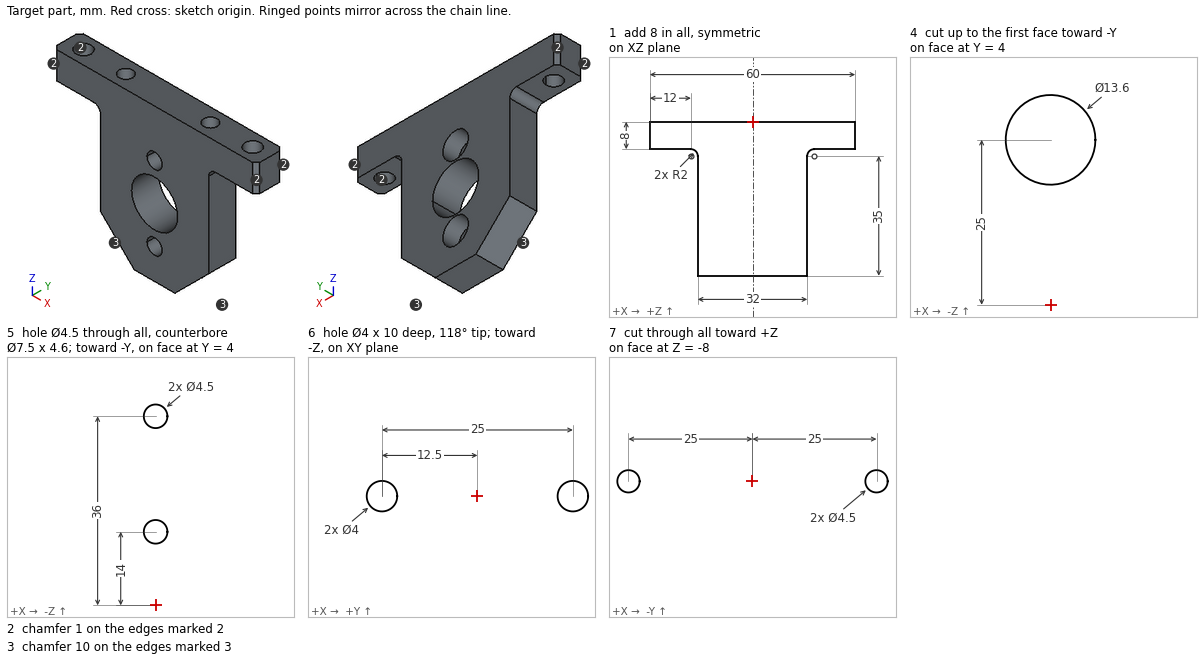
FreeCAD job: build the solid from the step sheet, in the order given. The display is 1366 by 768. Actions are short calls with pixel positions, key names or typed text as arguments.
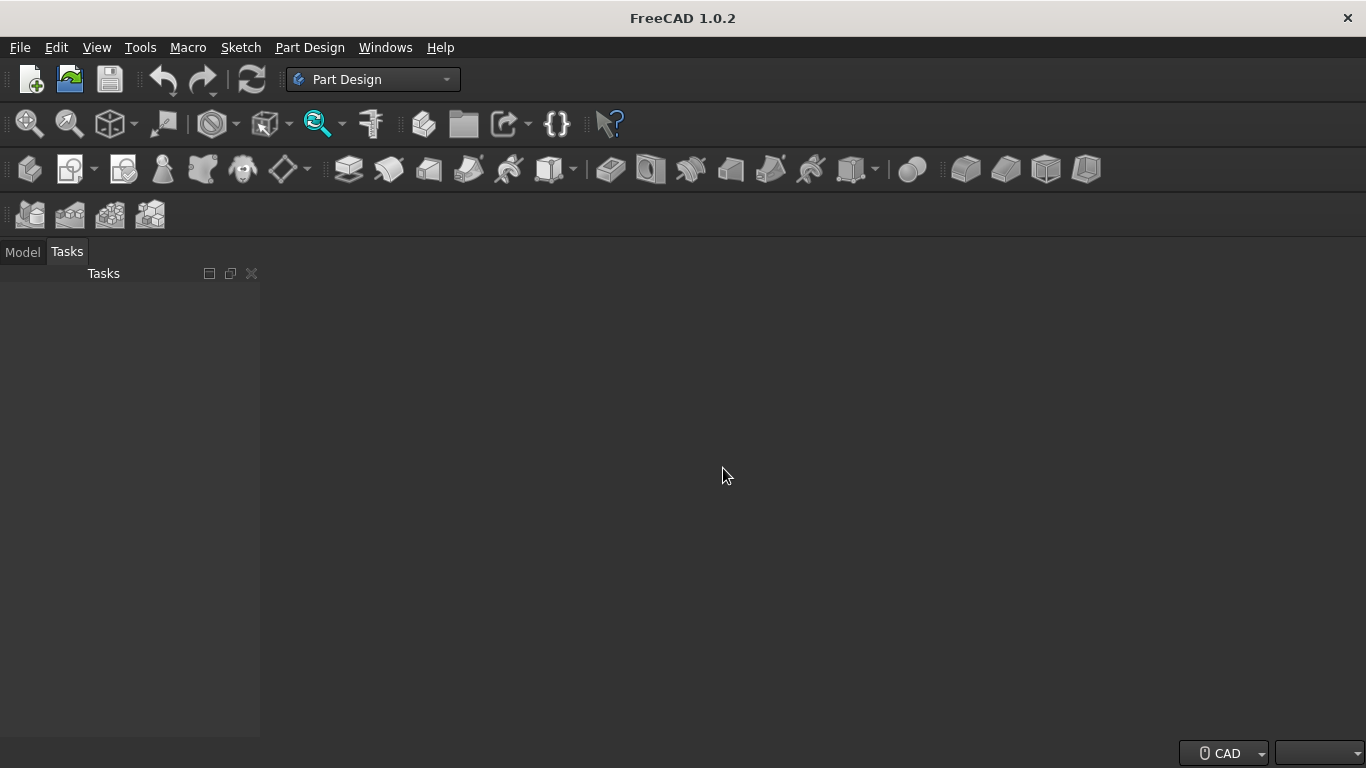
key(ctrl+n)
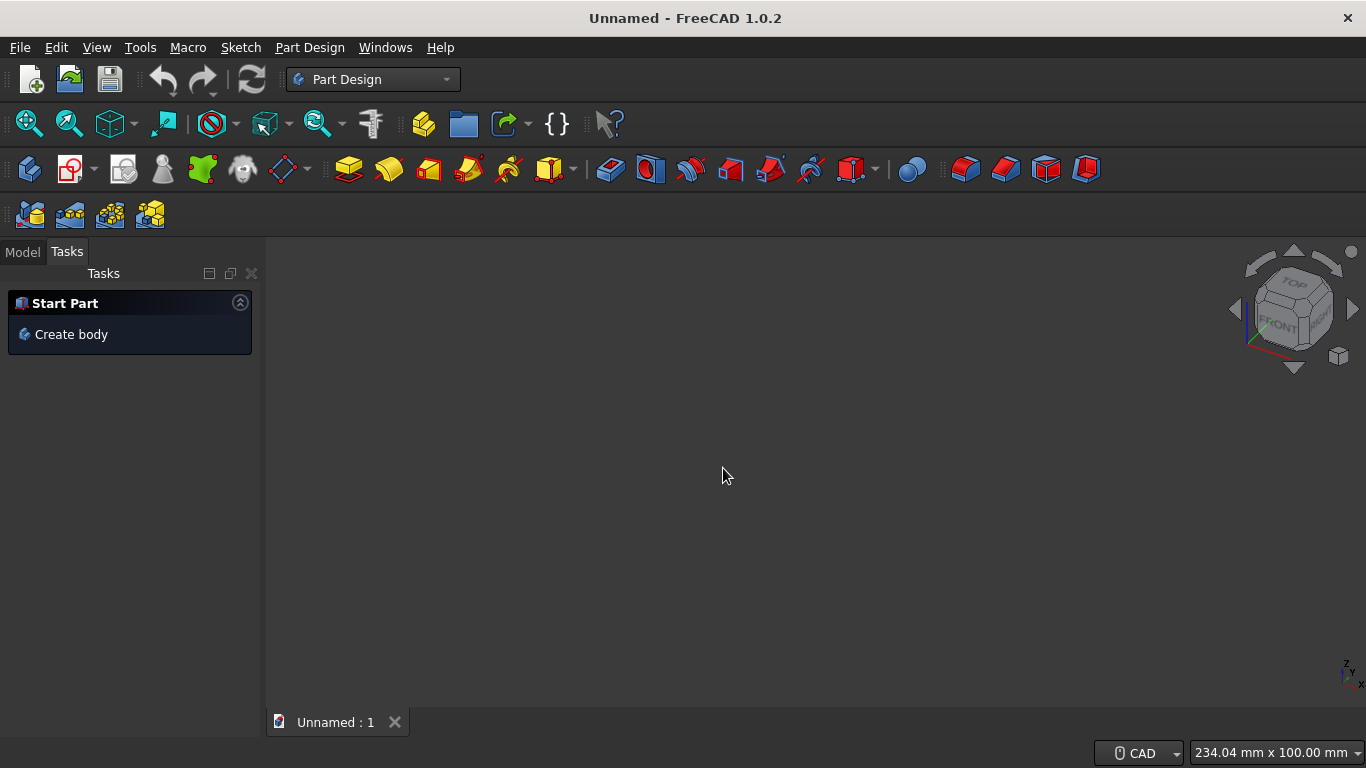
click(70, 170)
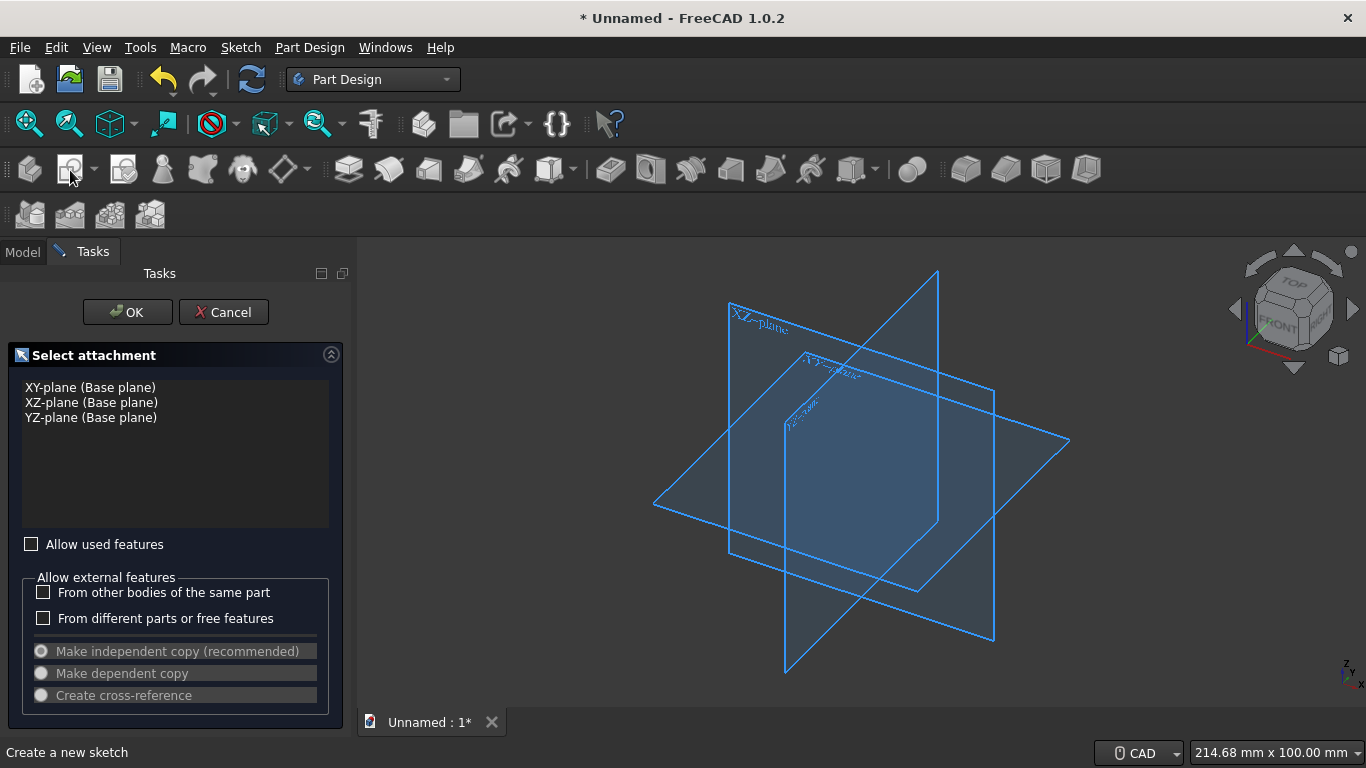
click(82, 402)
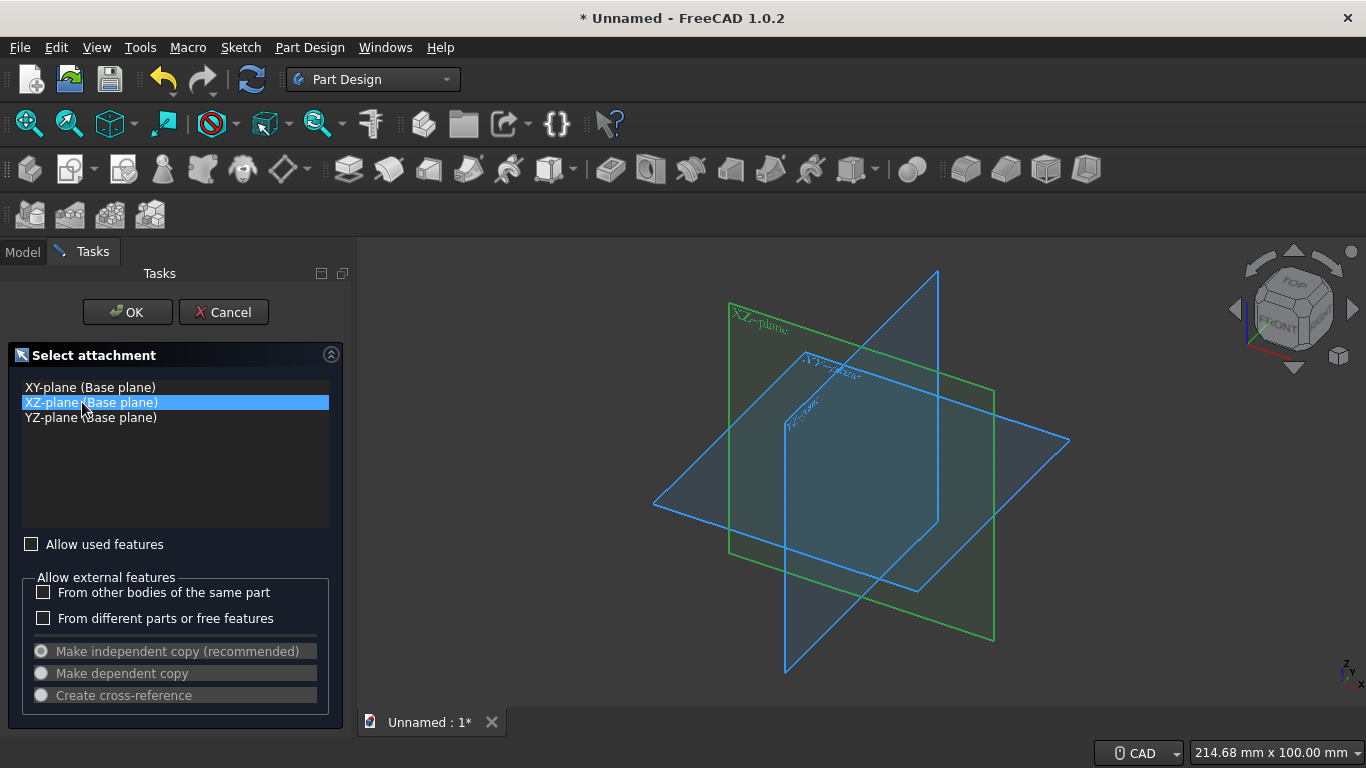
click(128, 312)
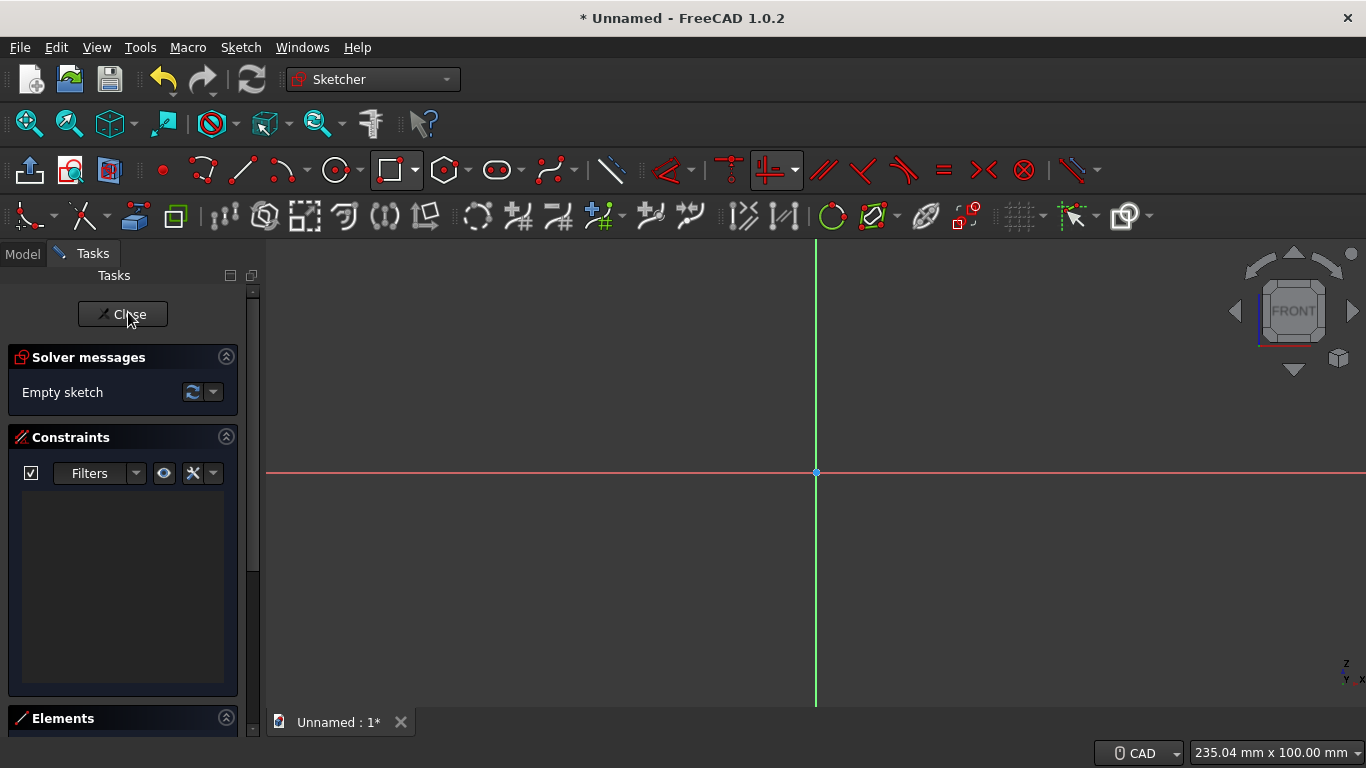
scroll(438, 267, down, 1)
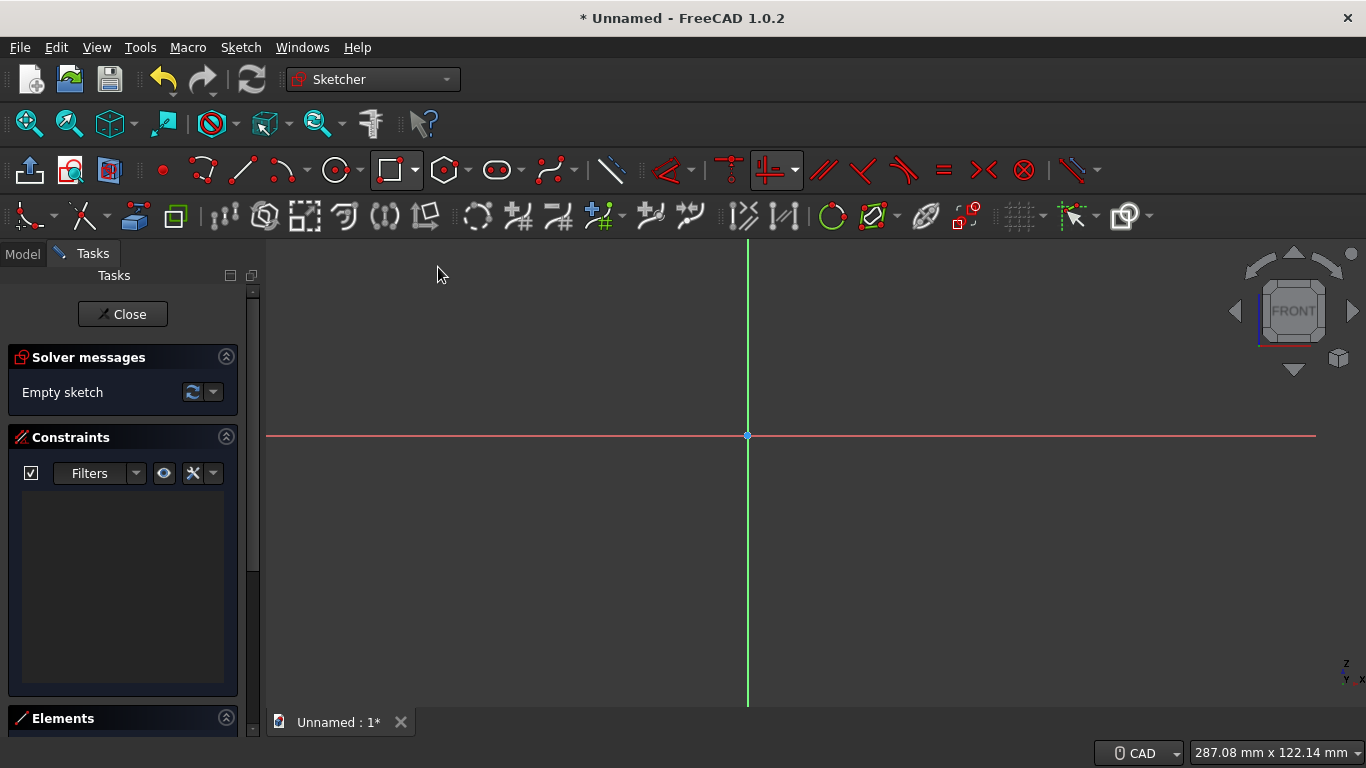
scroll(748, 581, up, 3)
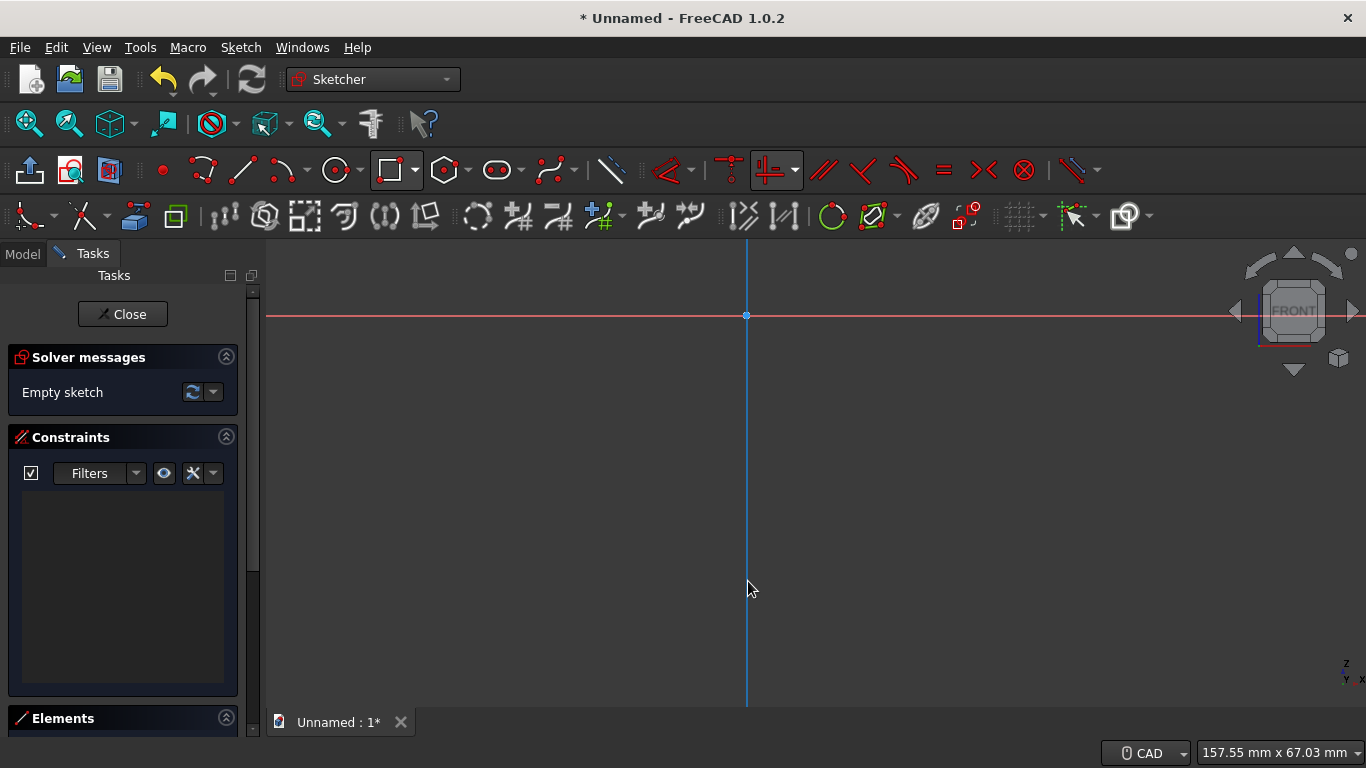
key(g)
key(m)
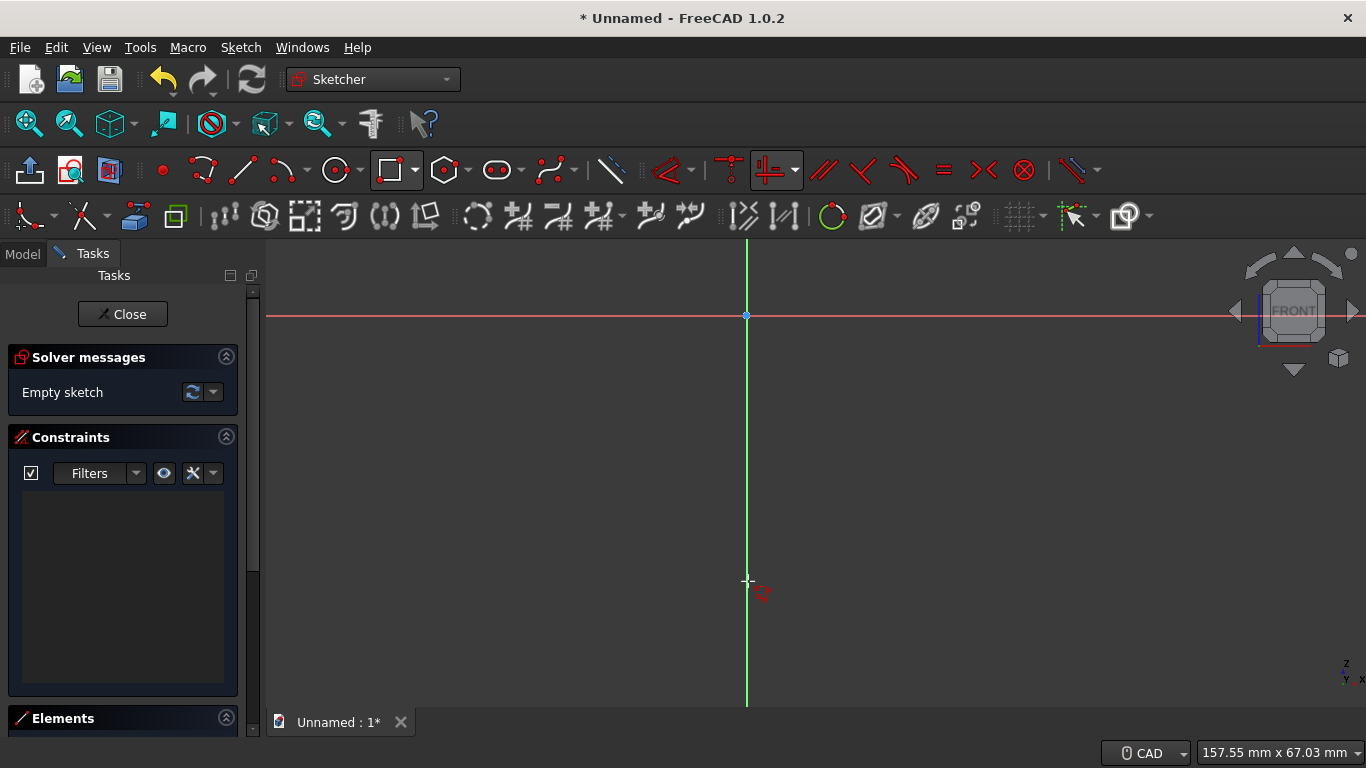
click(858, 385)
click(858, 630)
click(635, 630)
click(635, 385)
right_click(635, 385)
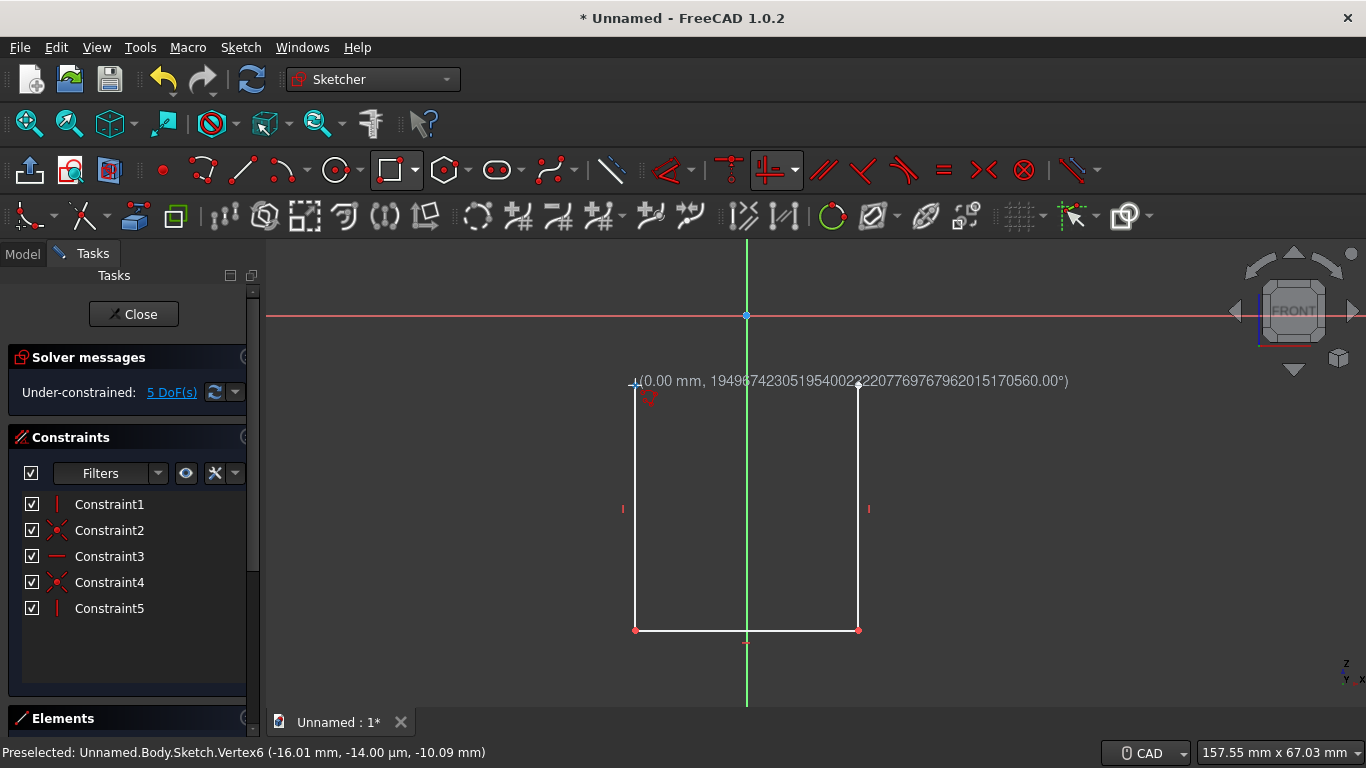
click(621, 371)
click(537, 371)
click(537, 316)
click(956, 325)
click(956, 371)
click(872, 371)
right_click(872, 371)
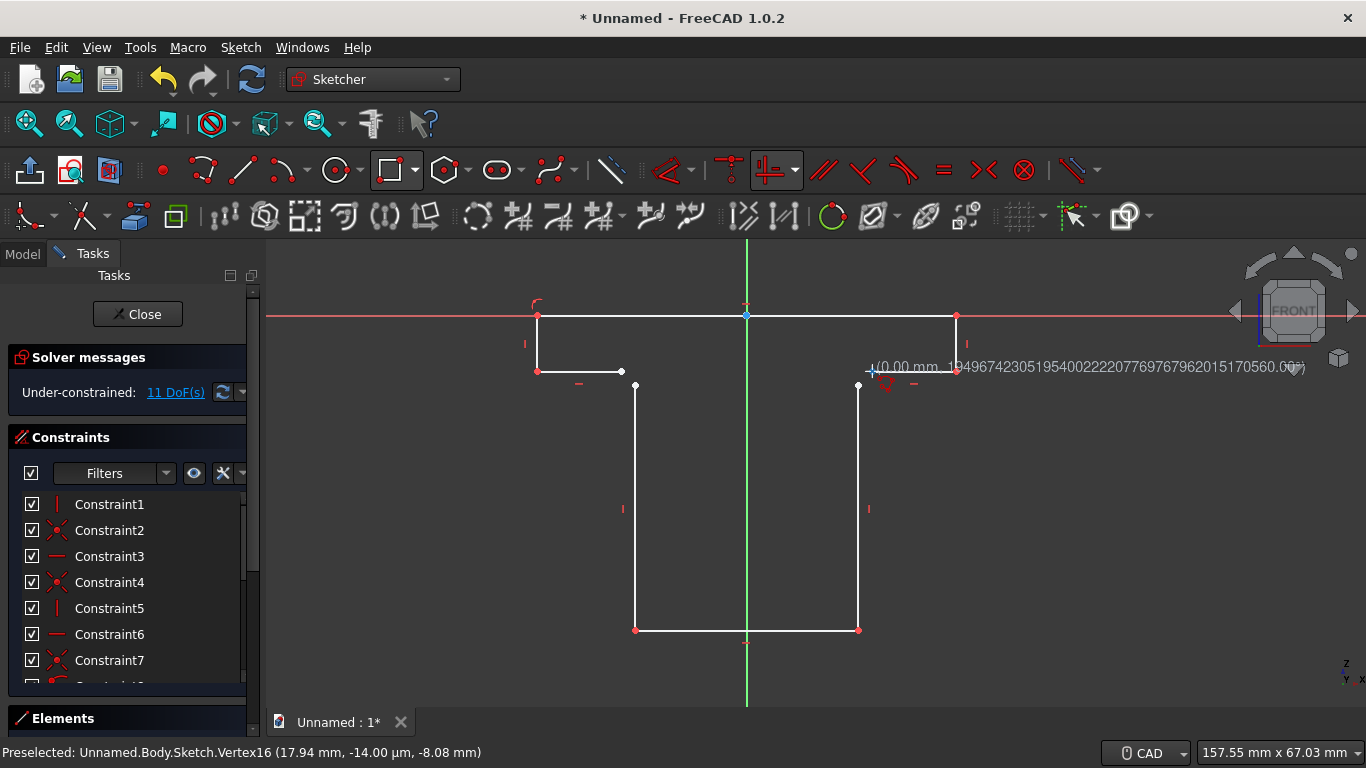
click(310, 170)